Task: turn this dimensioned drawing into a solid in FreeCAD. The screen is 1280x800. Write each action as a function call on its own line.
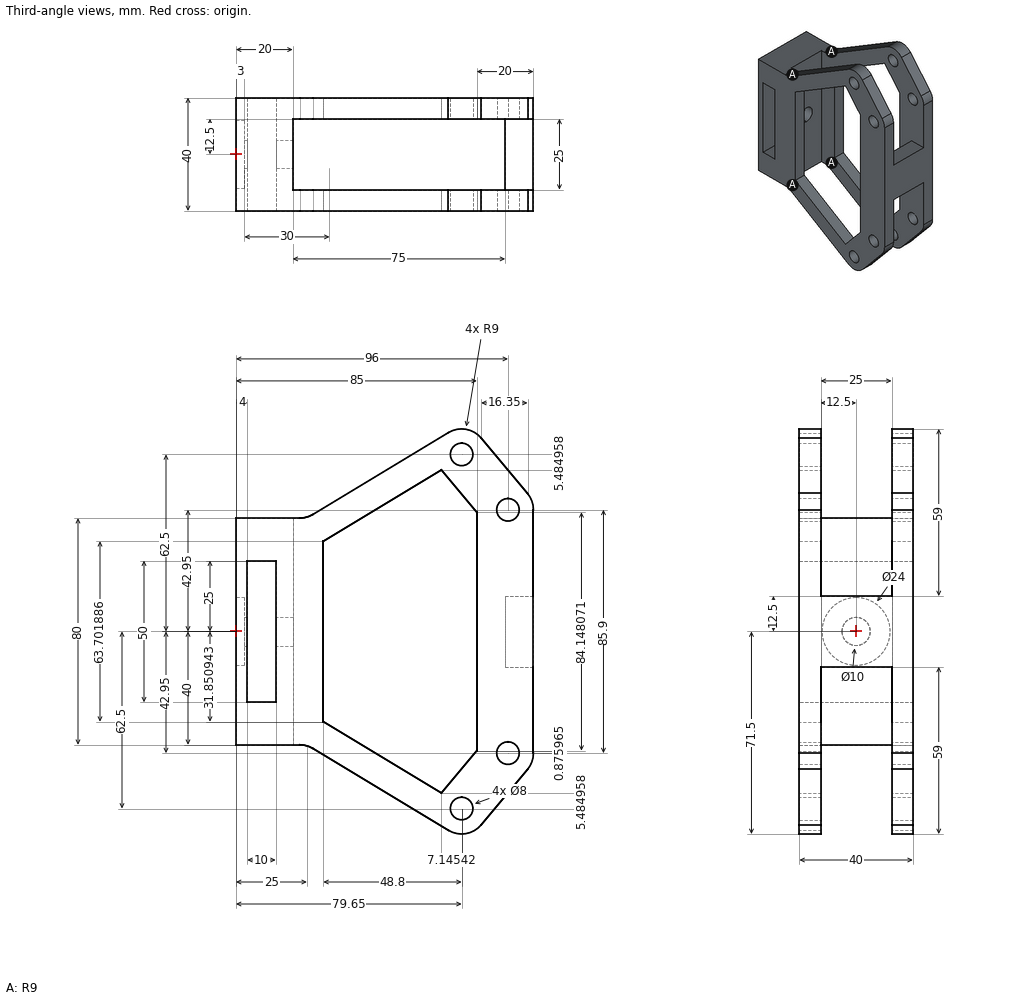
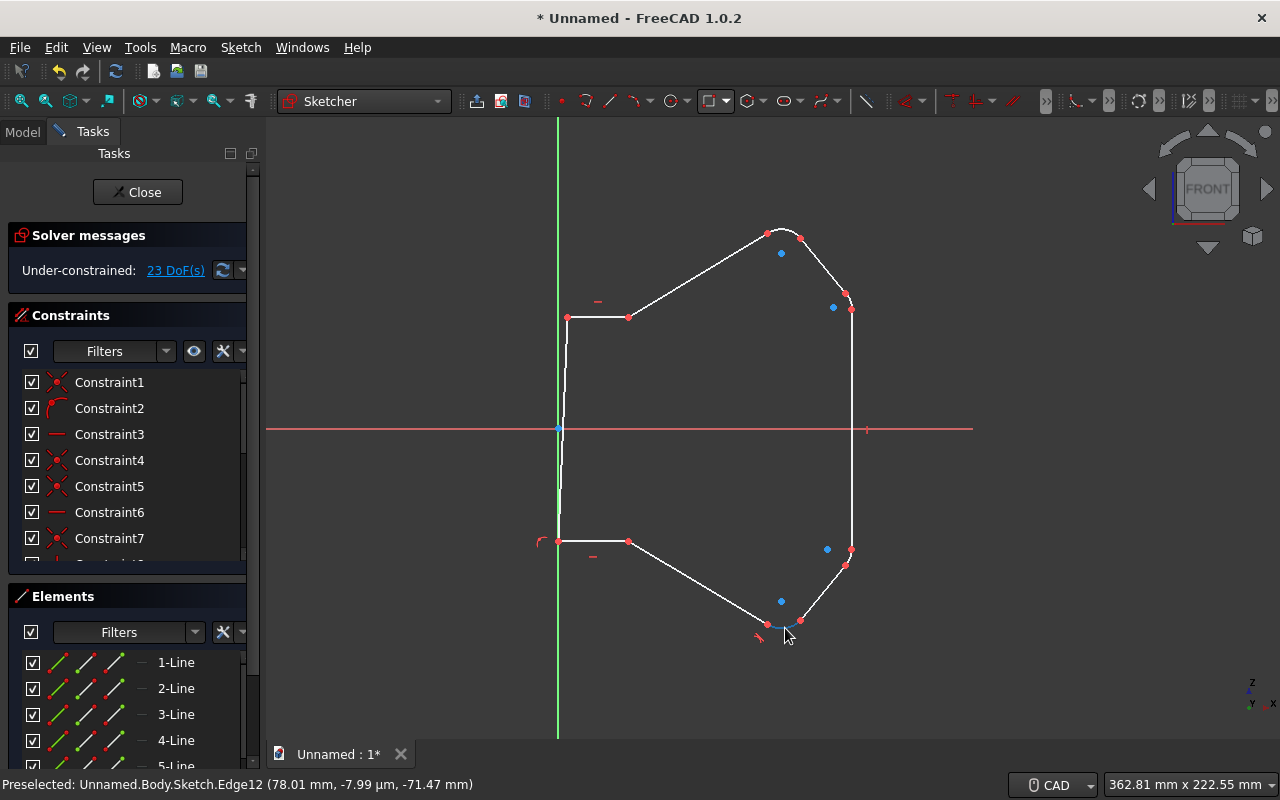
click(670, 292)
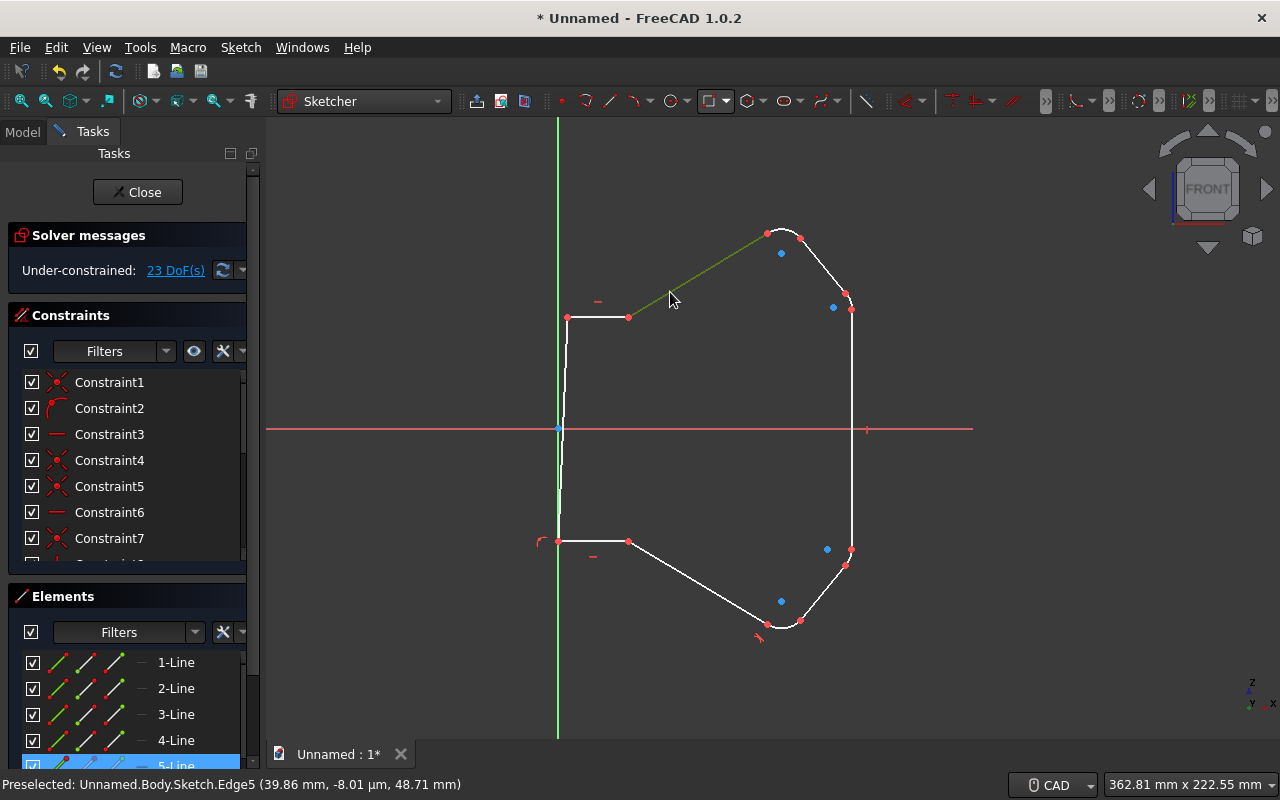
scroll(792, 232, up, 2)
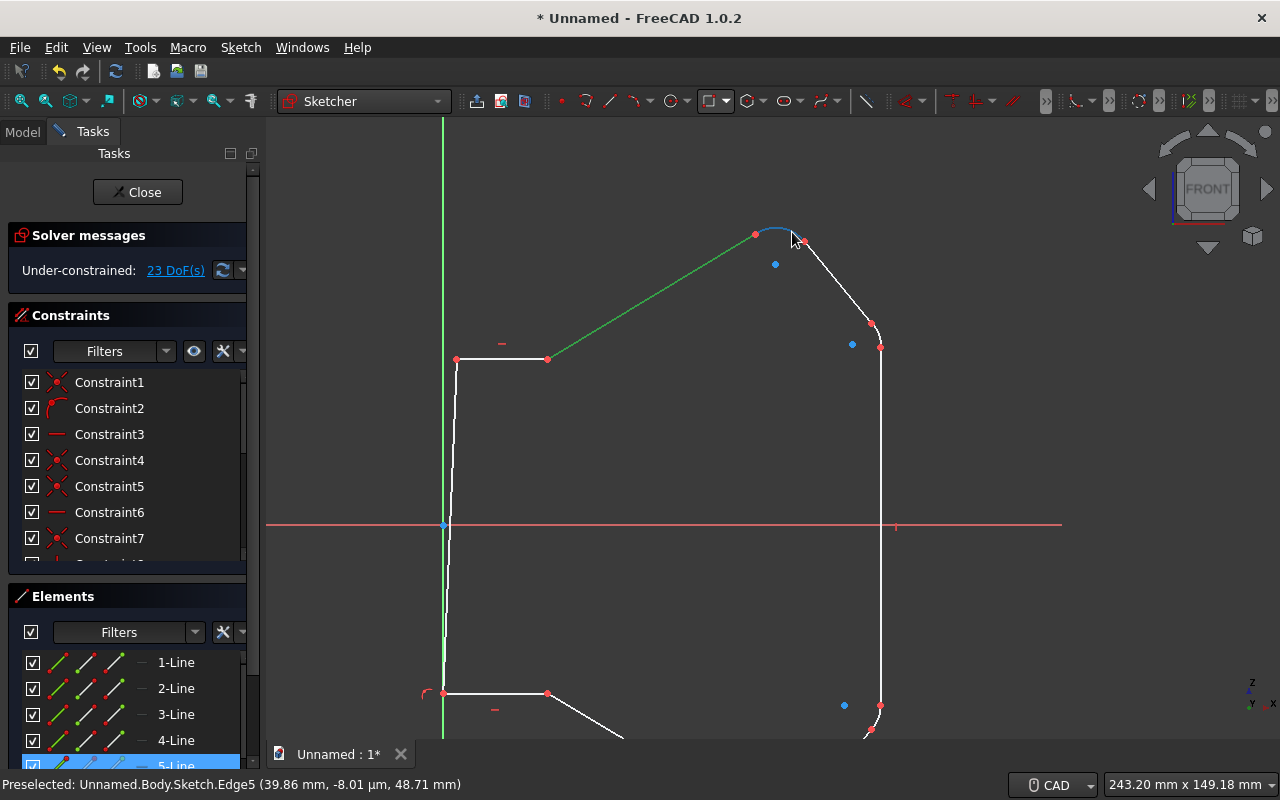
click(792, 231)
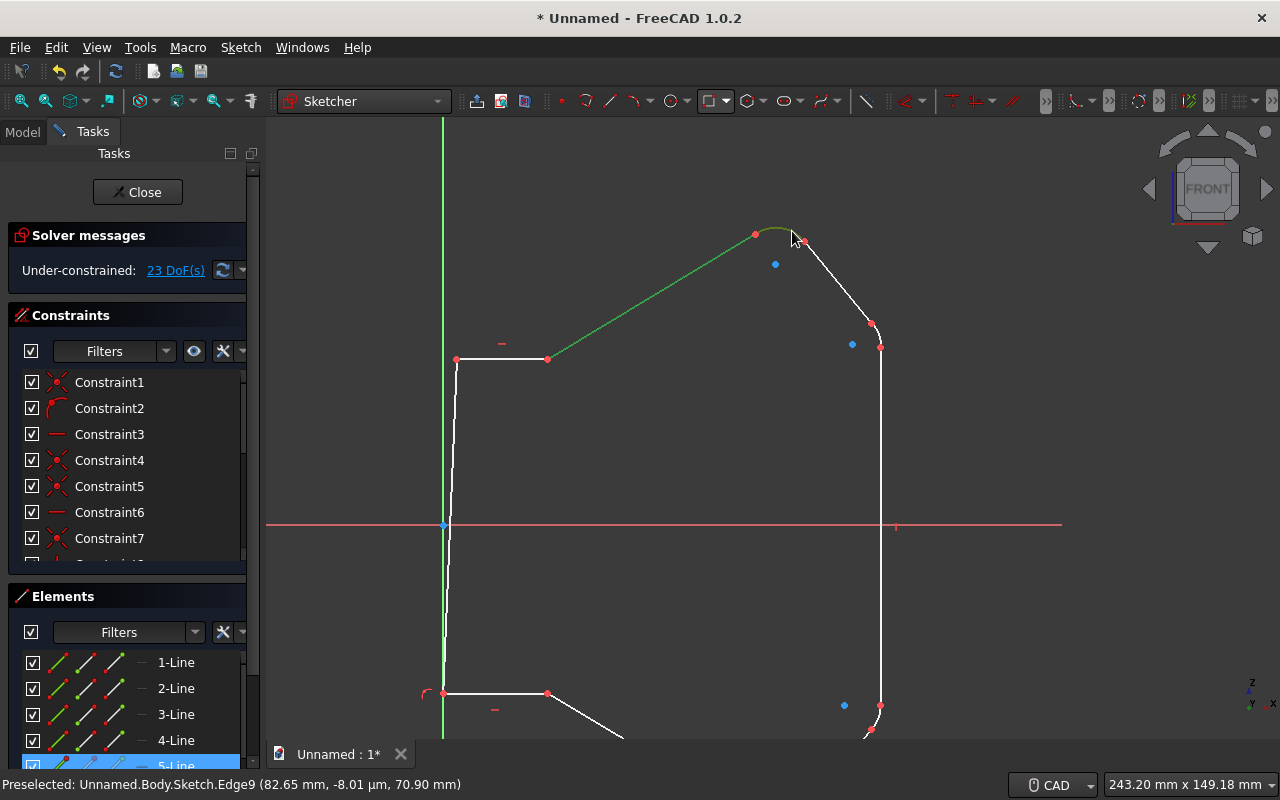
key(t)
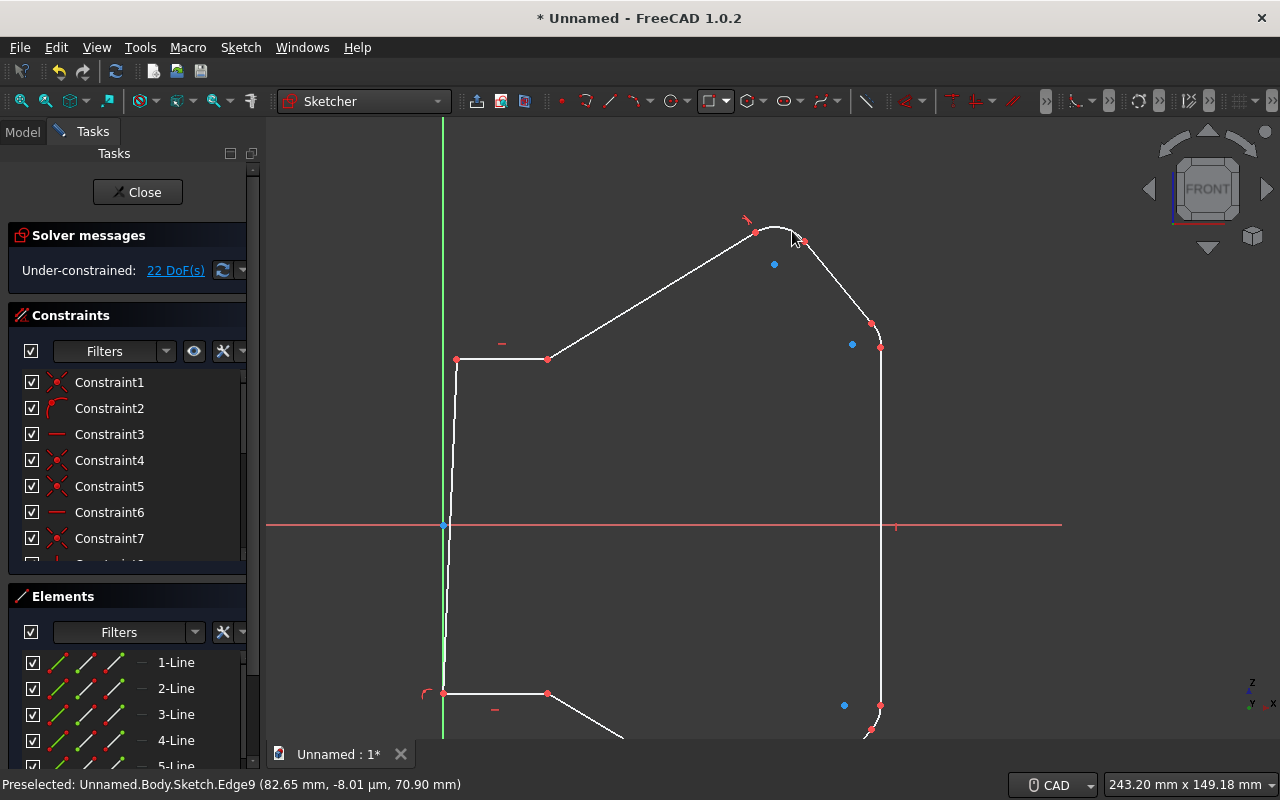
click(825, 266)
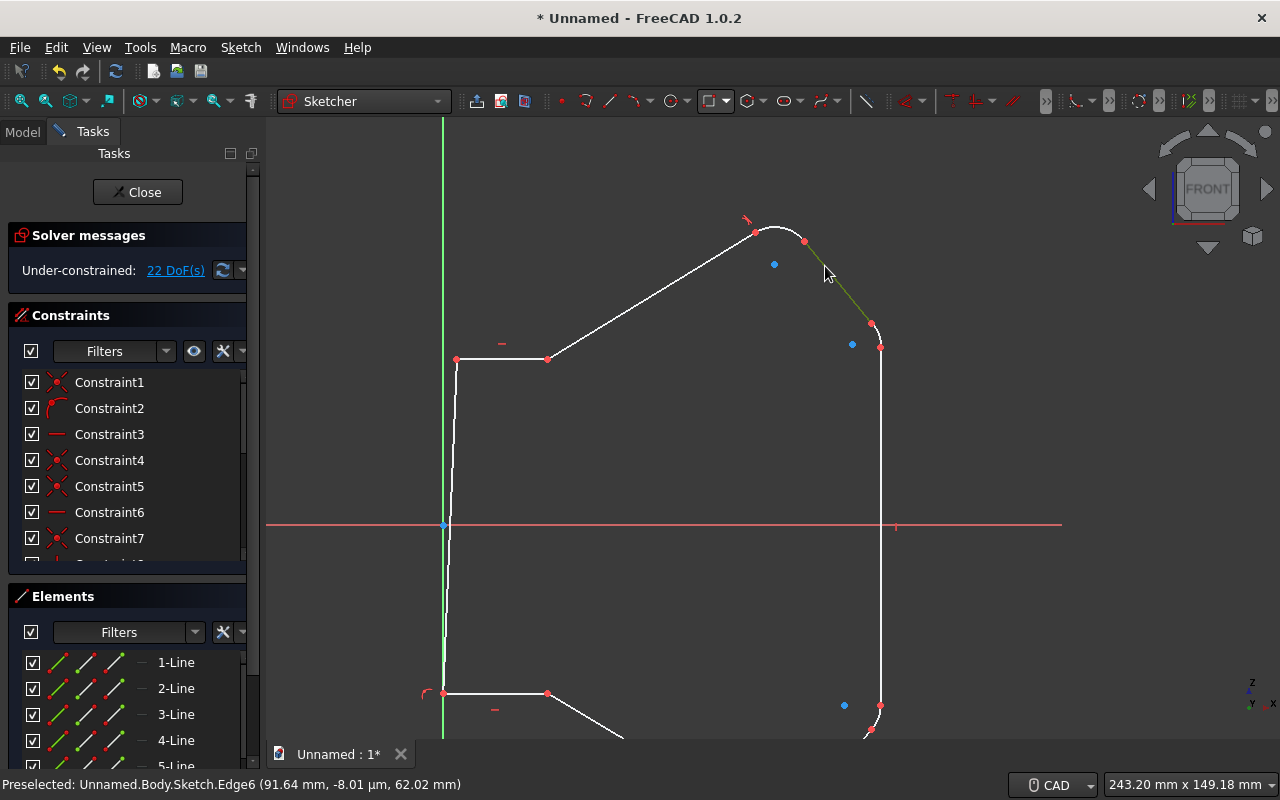
click(792, 231)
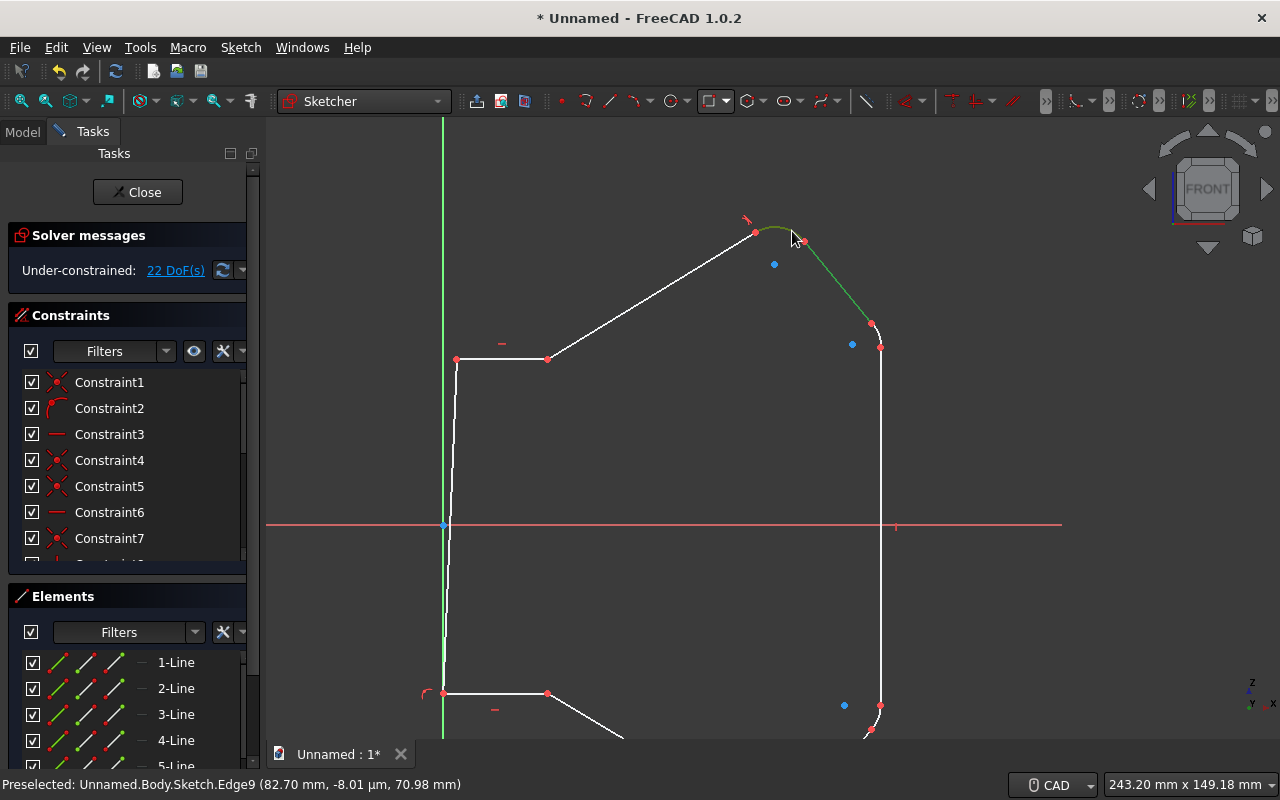
key(t)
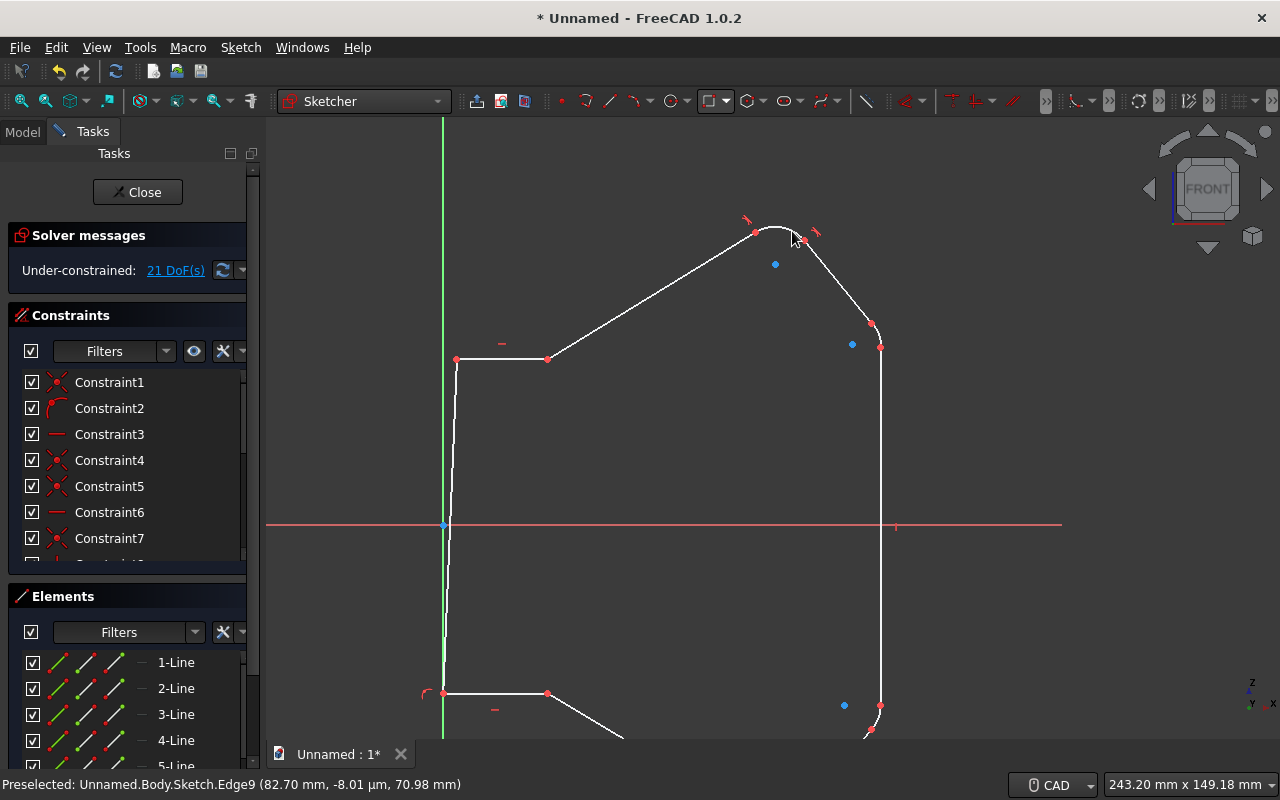
click(825, 266)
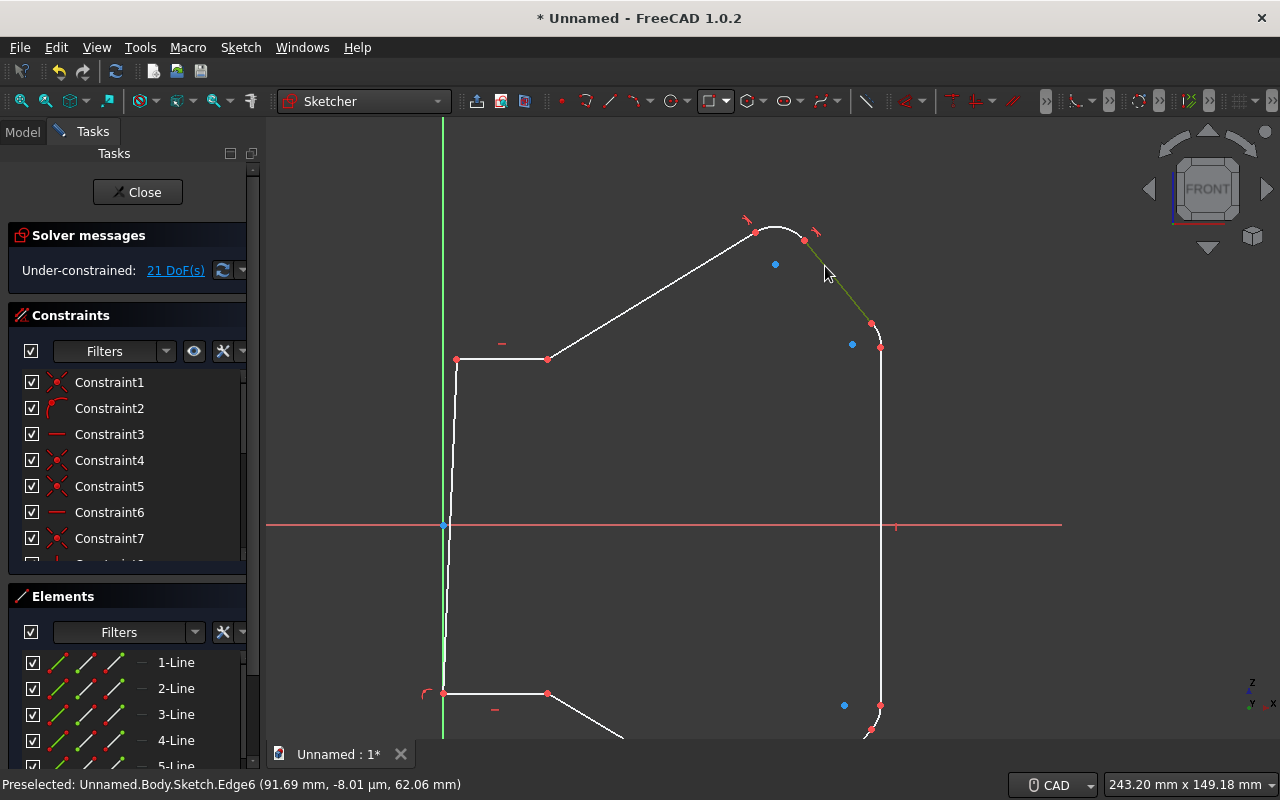
click(879, 334)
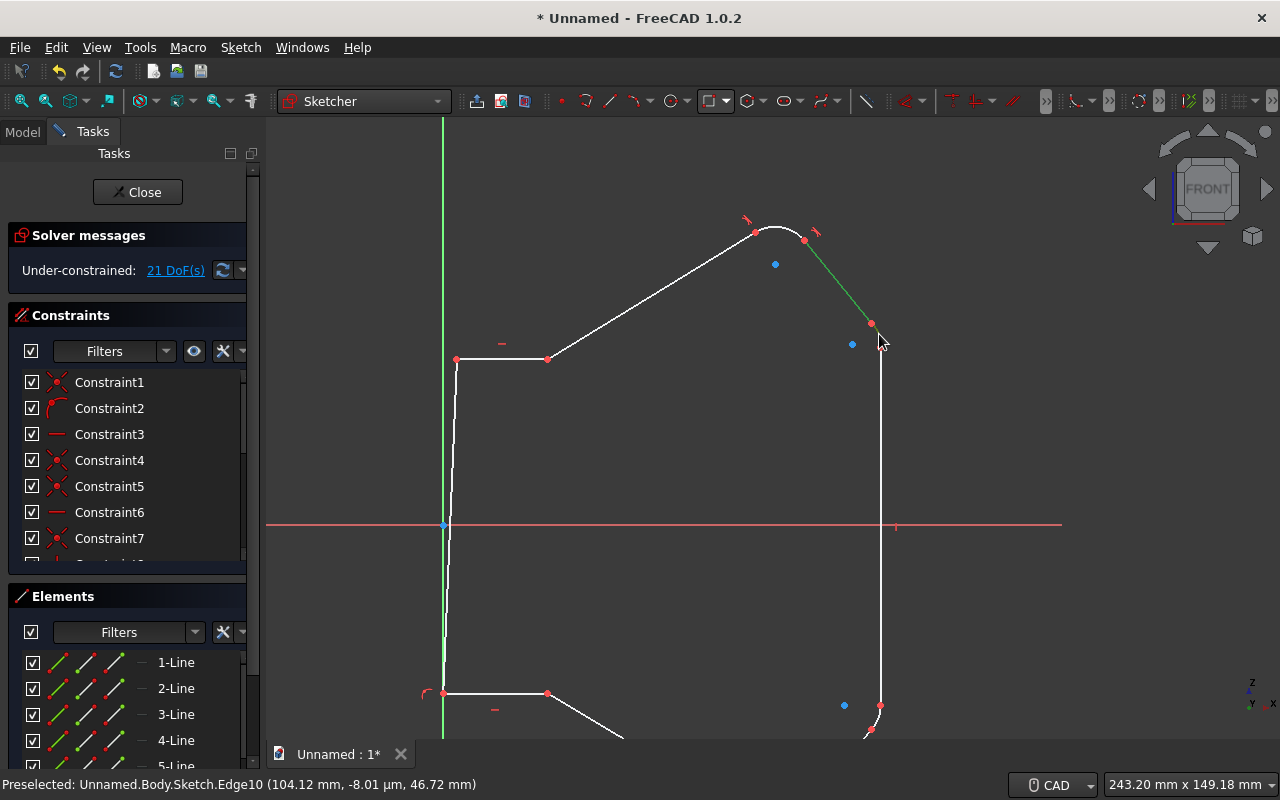
key(t)